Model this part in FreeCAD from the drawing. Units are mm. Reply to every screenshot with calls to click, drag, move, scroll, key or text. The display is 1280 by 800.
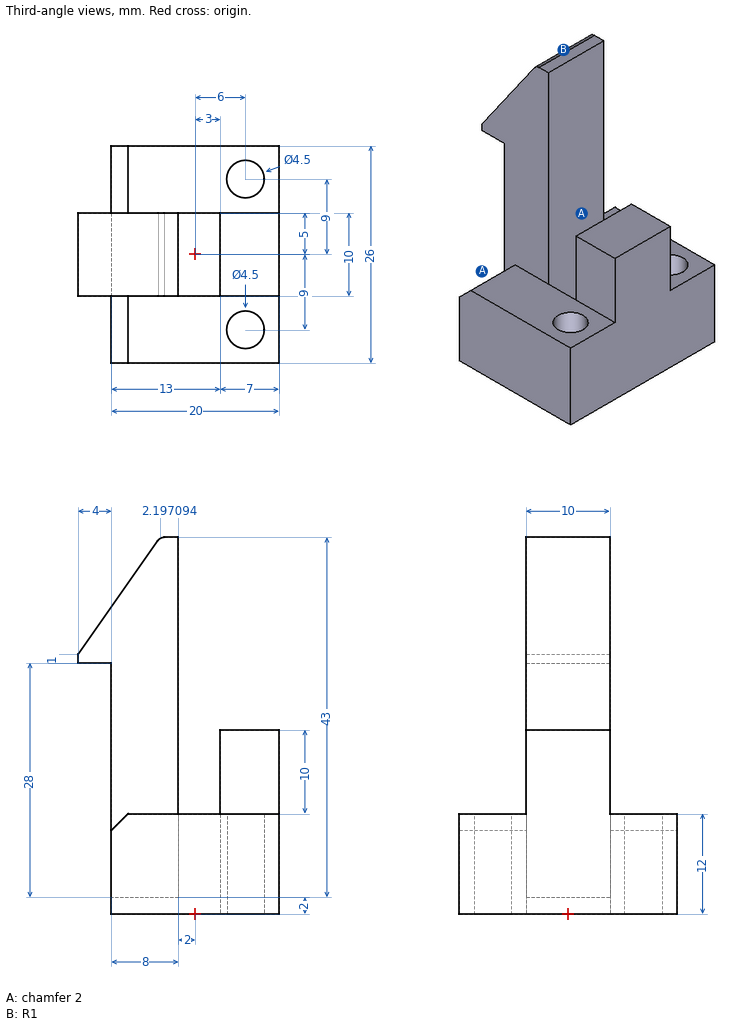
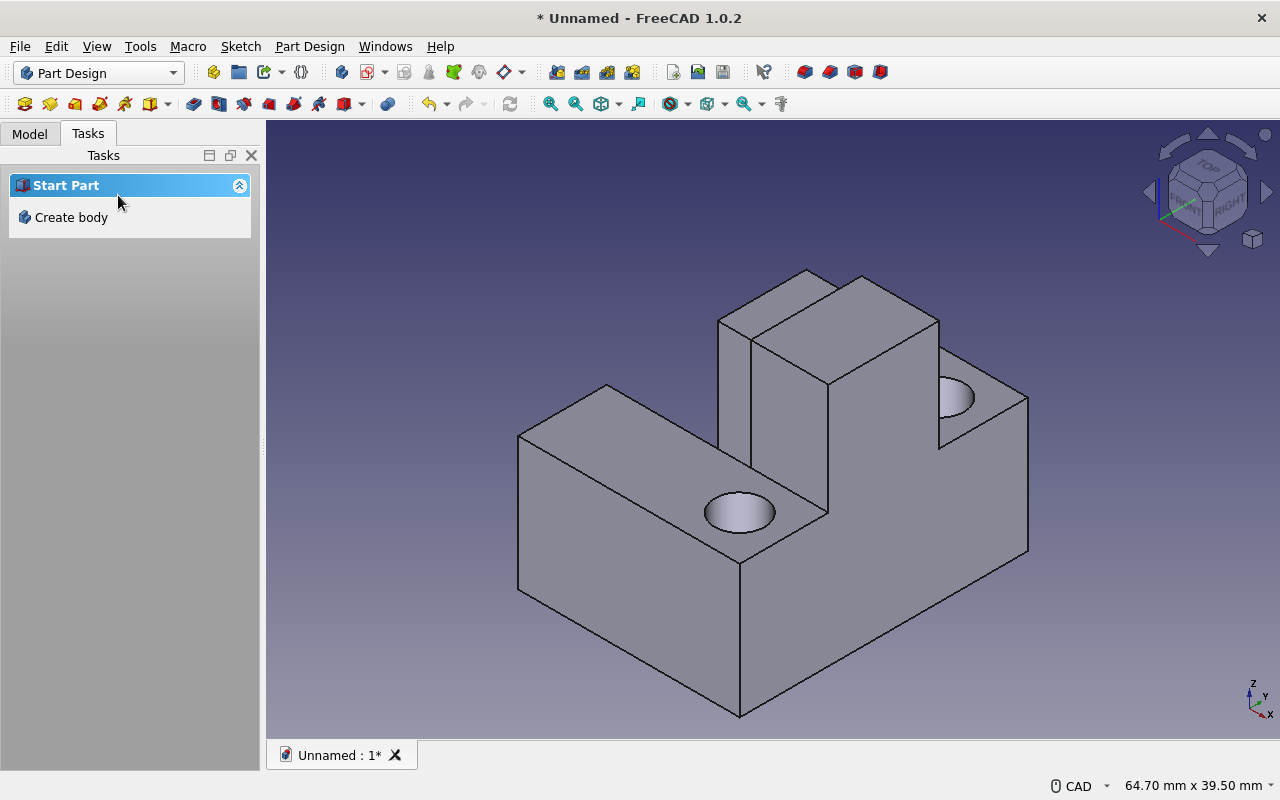
key(2)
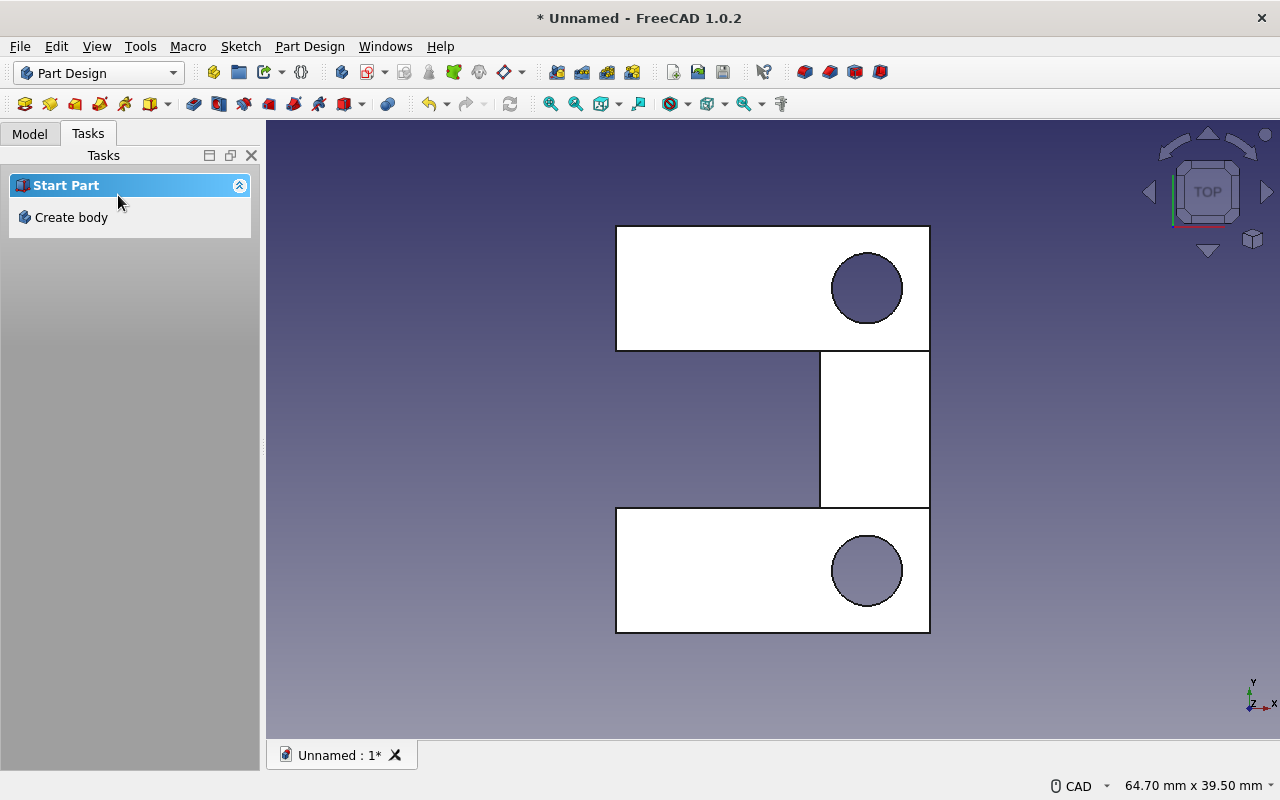
click(616, 570)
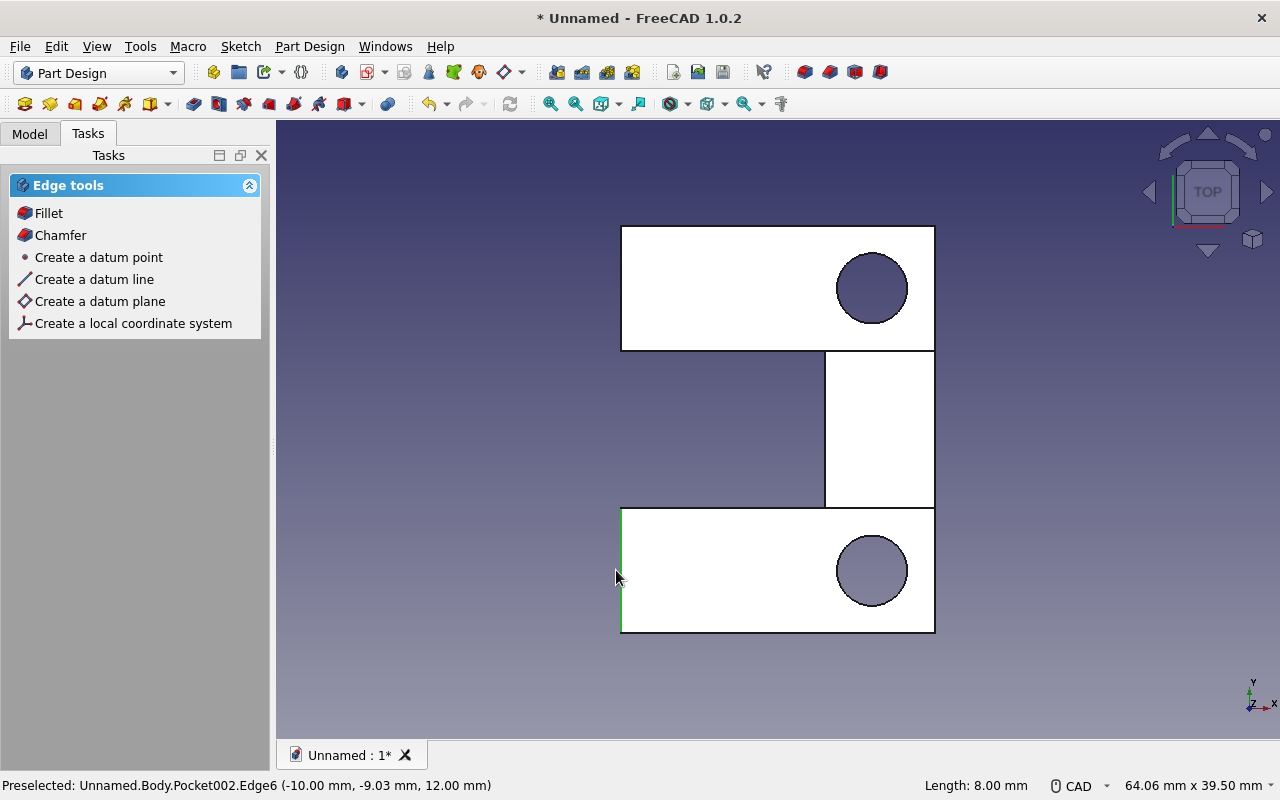
click(621, 287, ctrl)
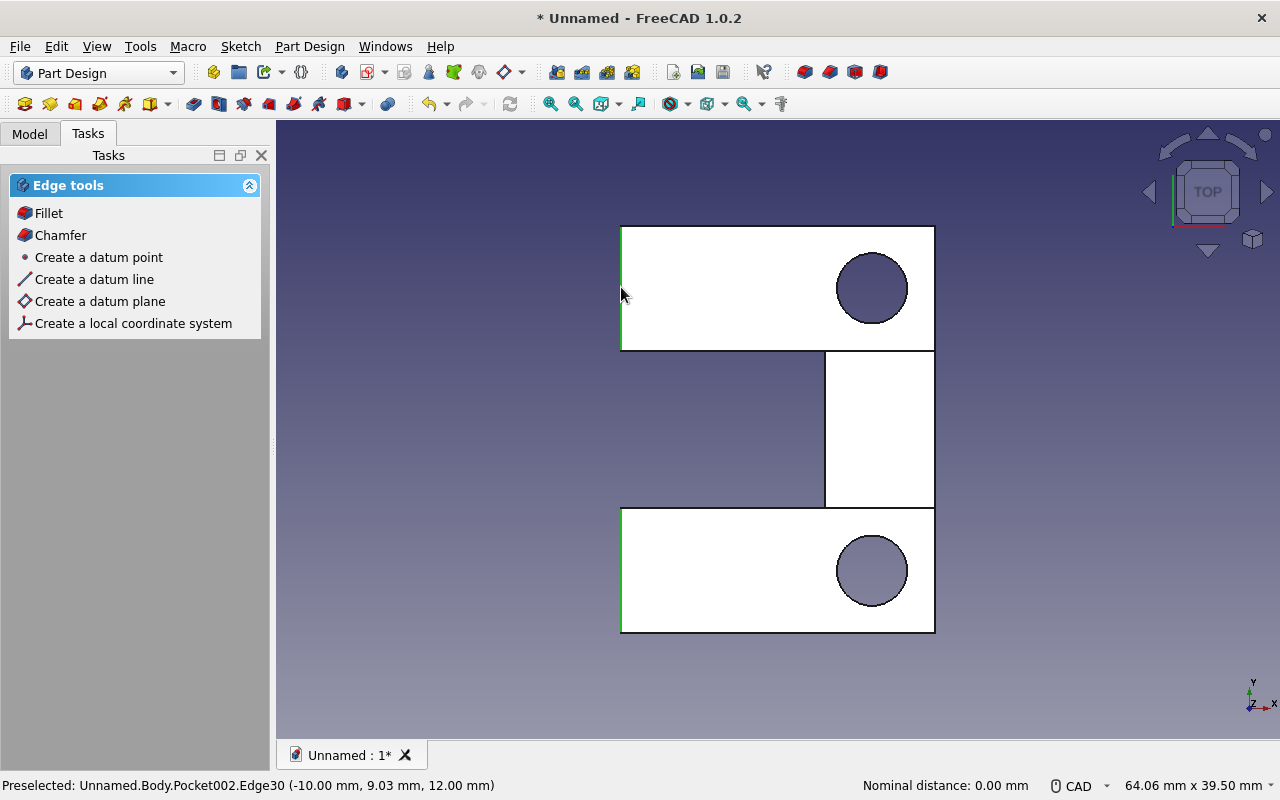
click(830, 72)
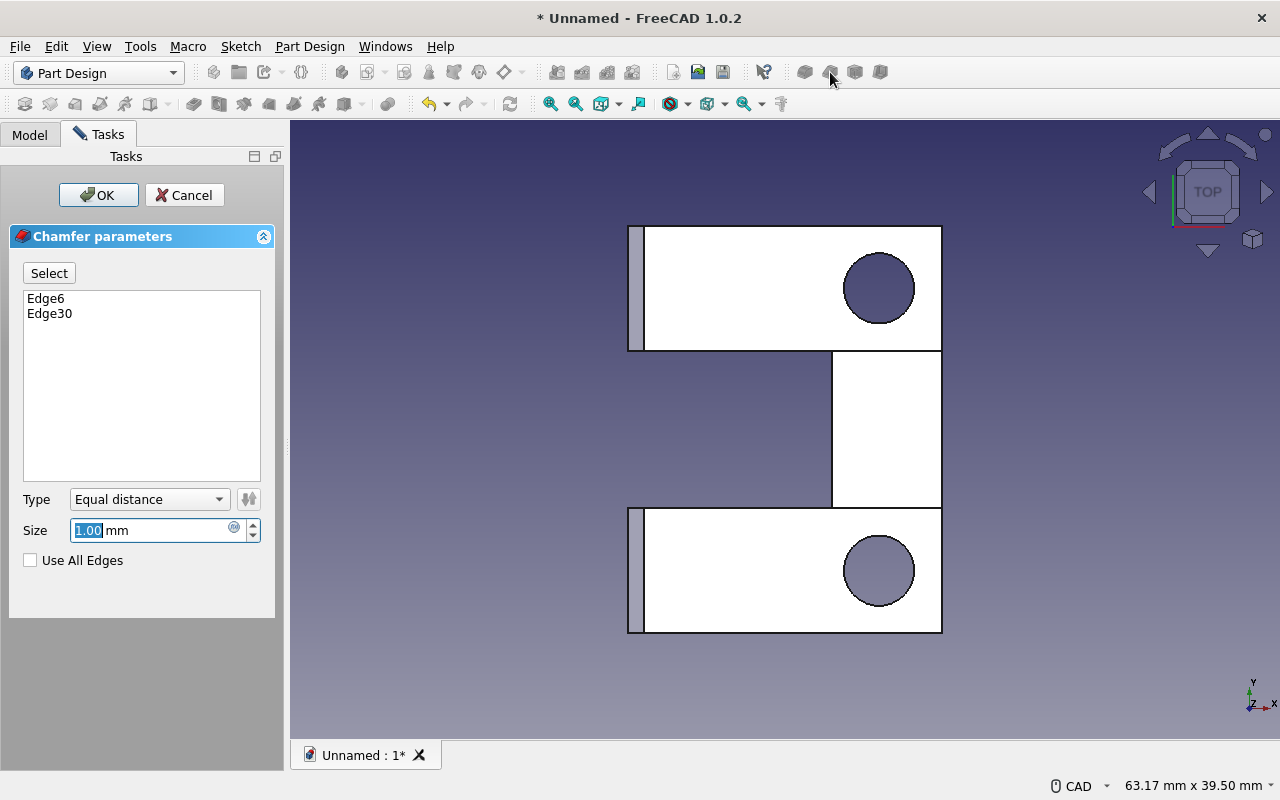
text(2)
key(Tab)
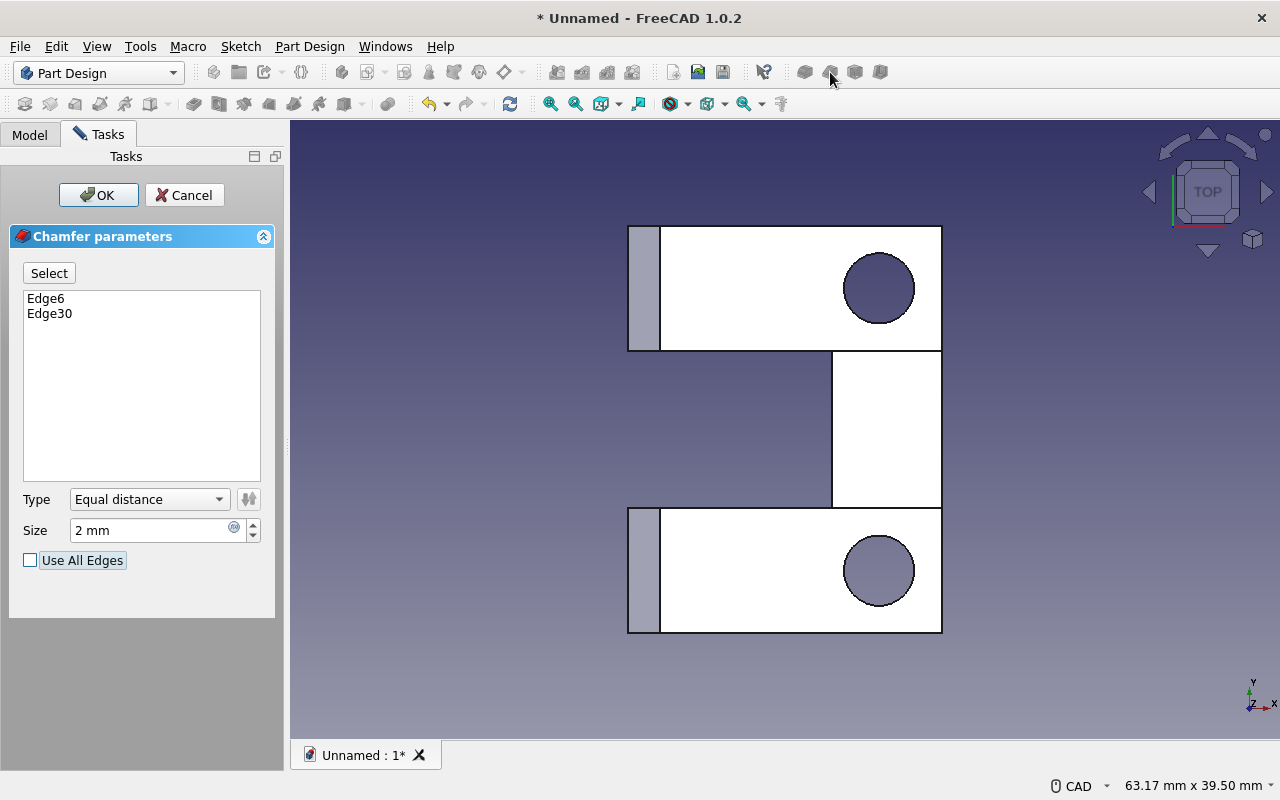
click(99, 195)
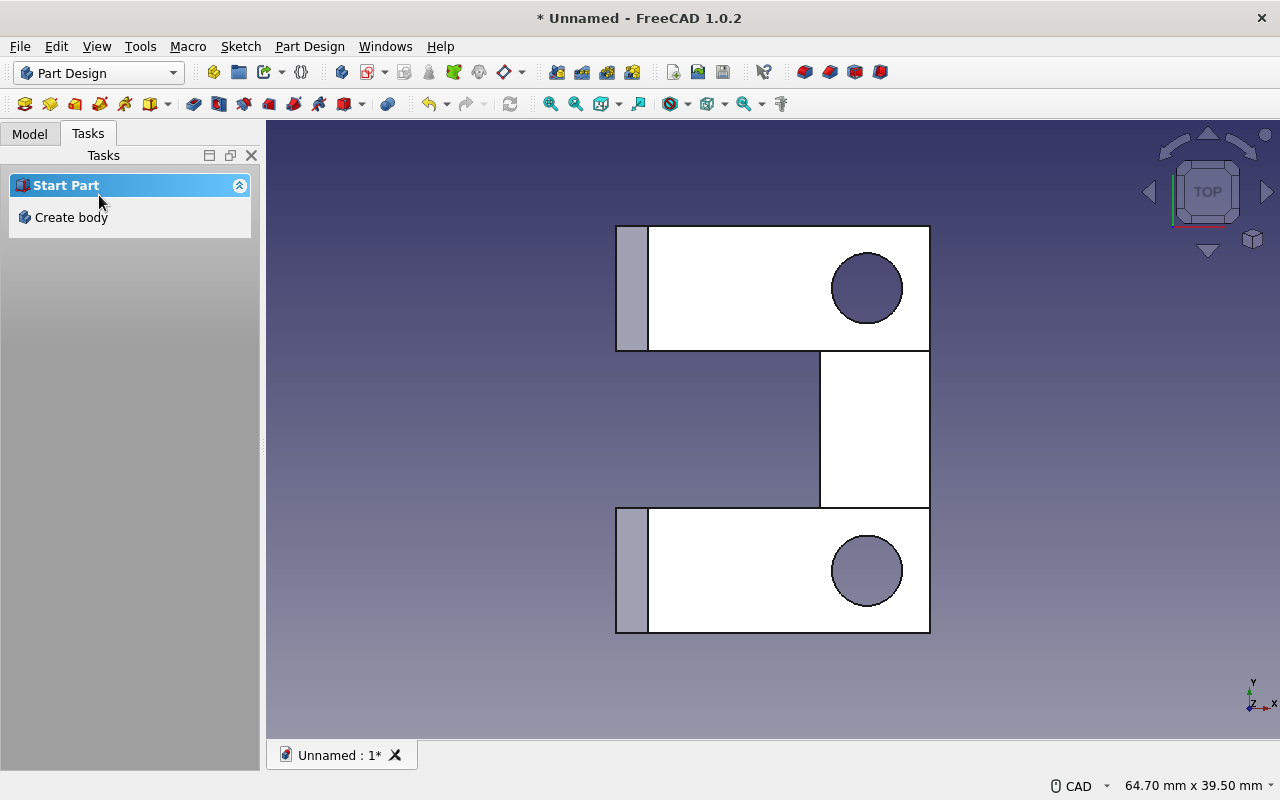
click(342, 72)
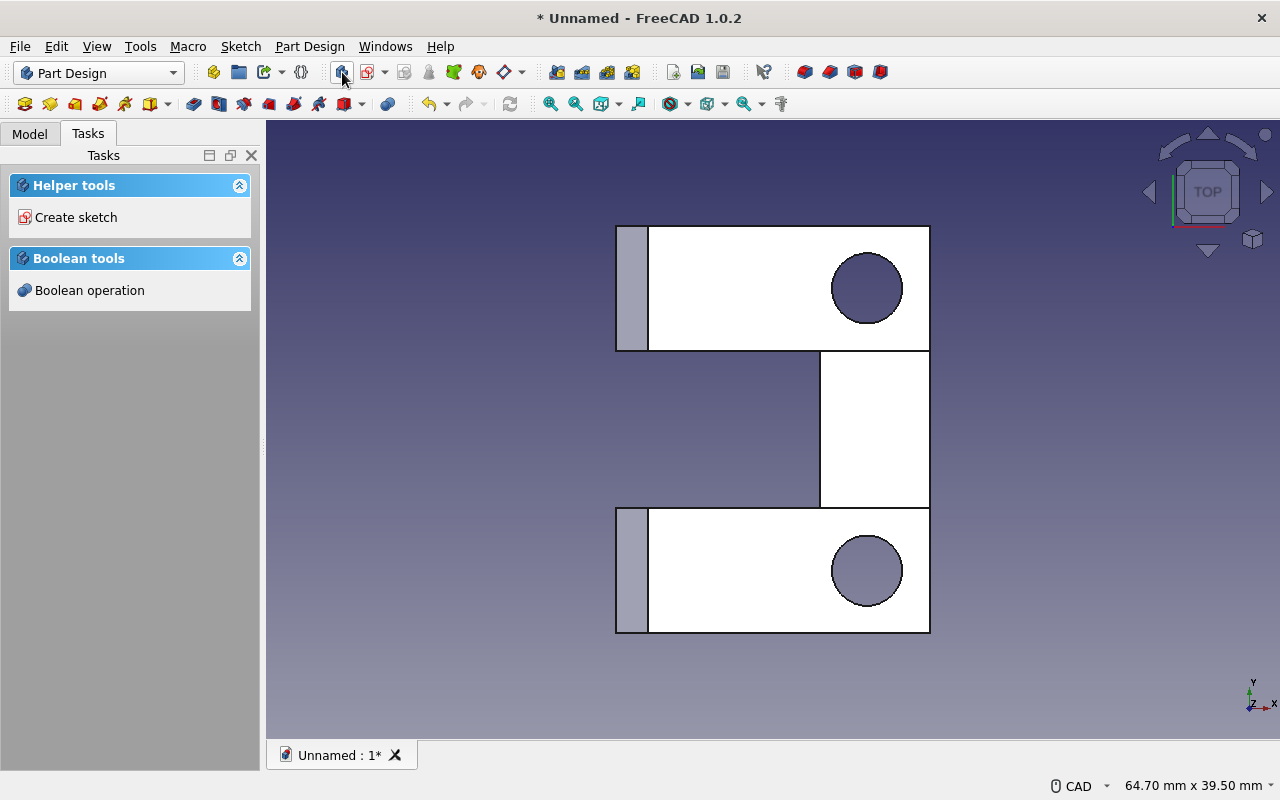
click(306, 699)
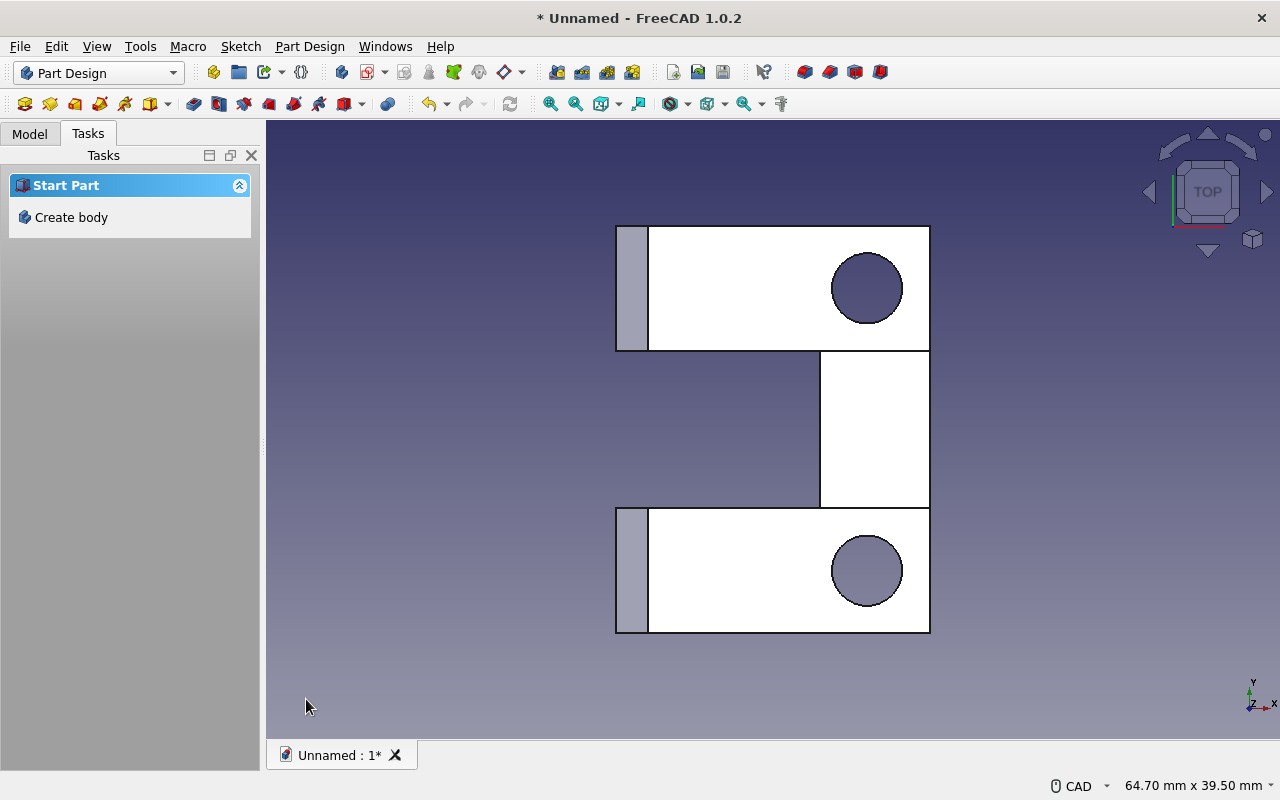
click(366, 72)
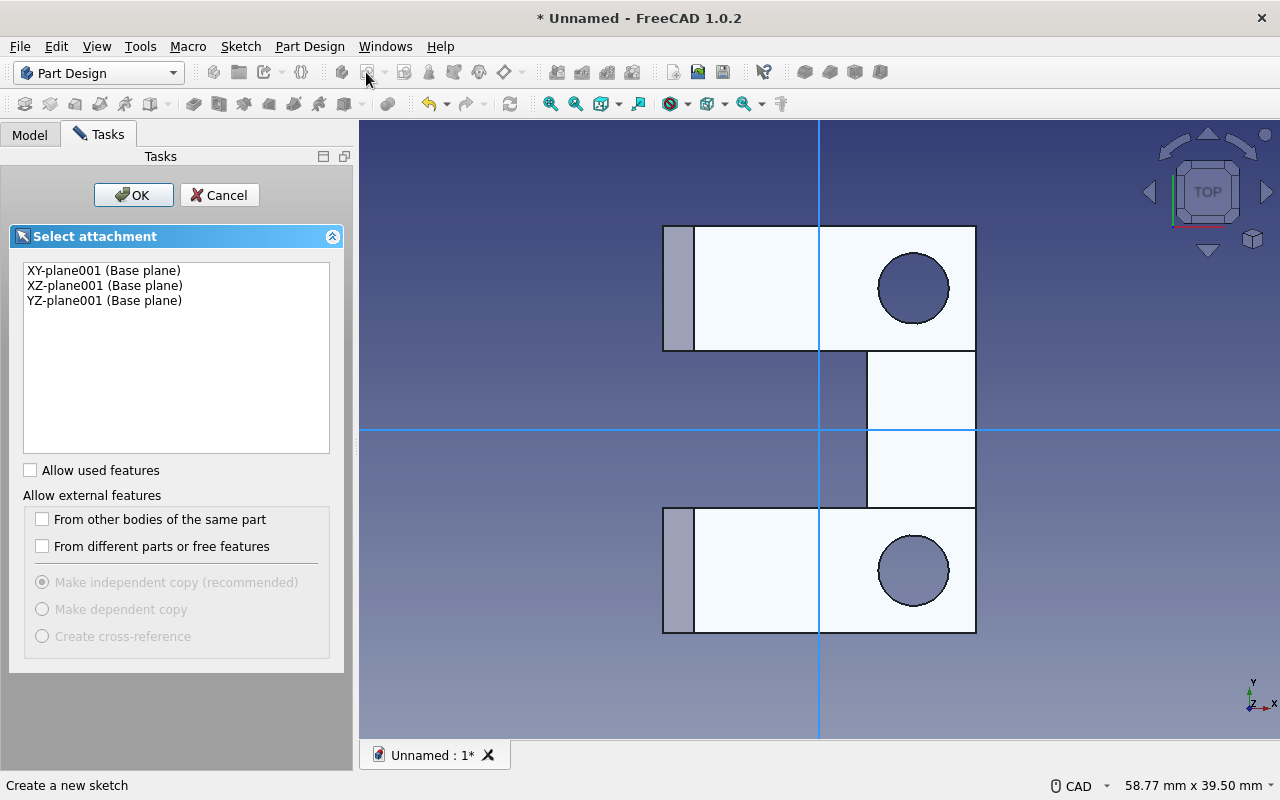
click(84, 286)